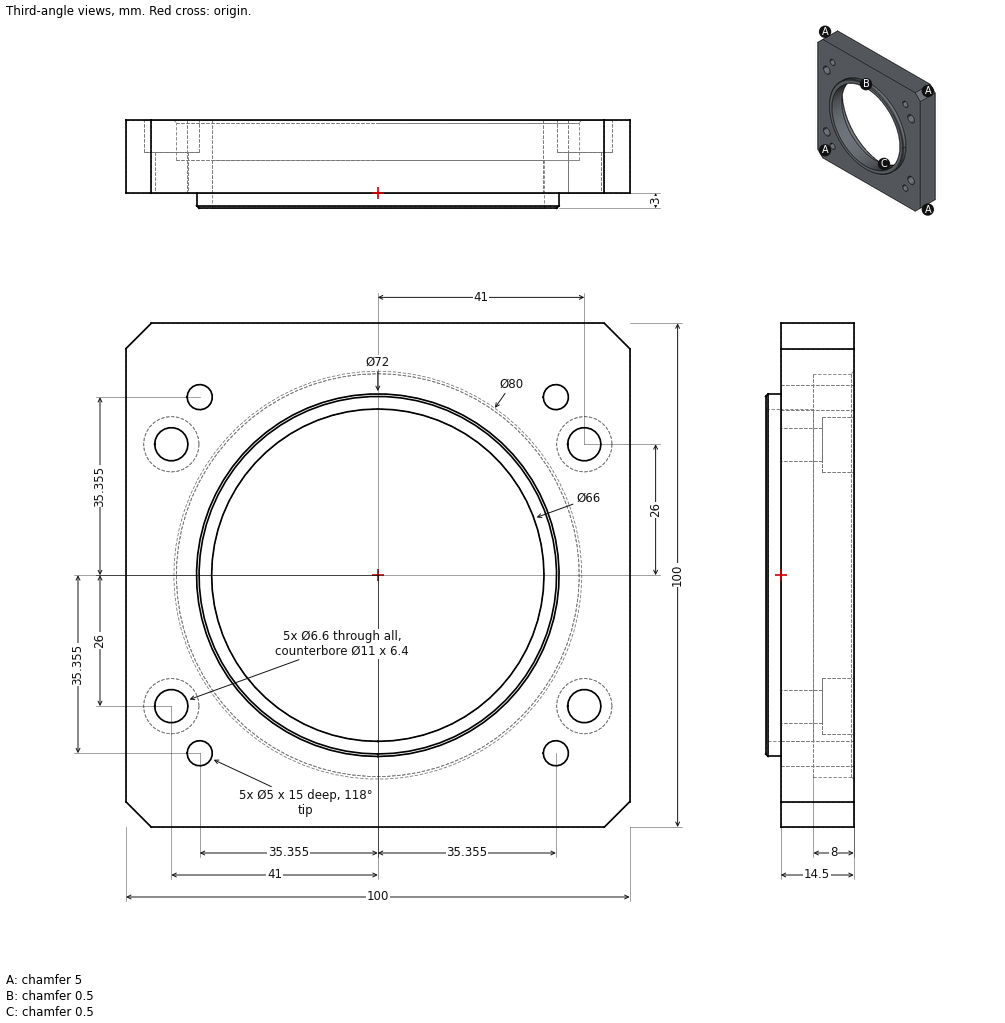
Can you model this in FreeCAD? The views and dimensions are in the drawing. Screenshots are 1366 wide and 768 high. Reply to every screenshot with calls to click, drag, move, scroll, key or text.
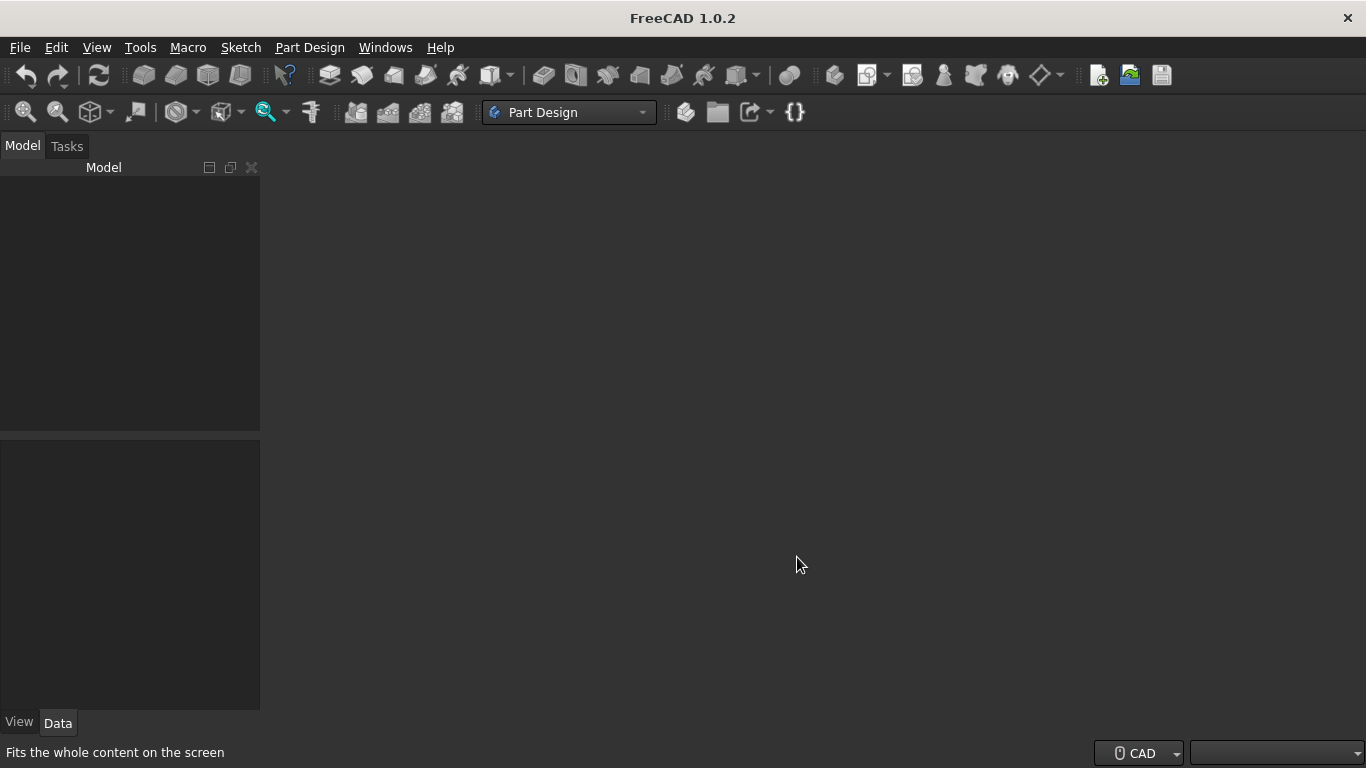
click(1098, 76)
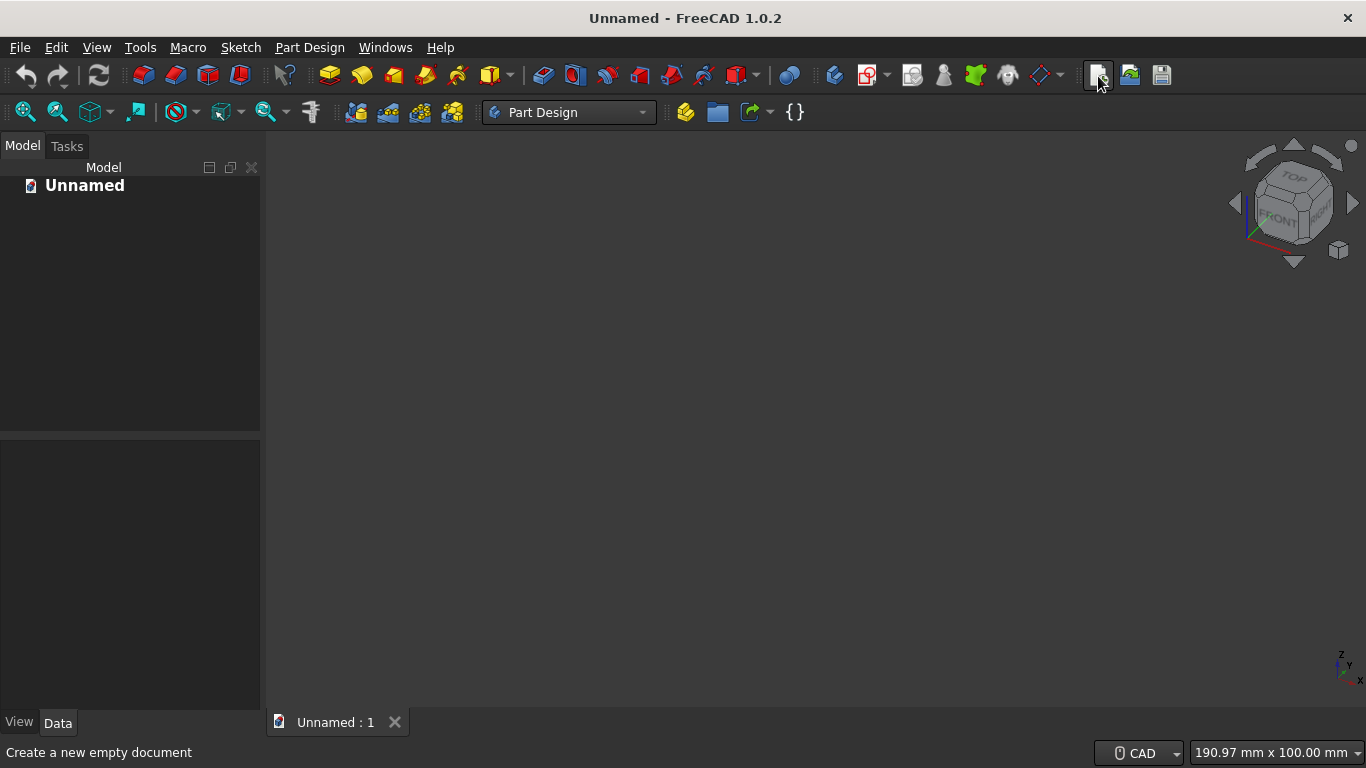
click(868, 76)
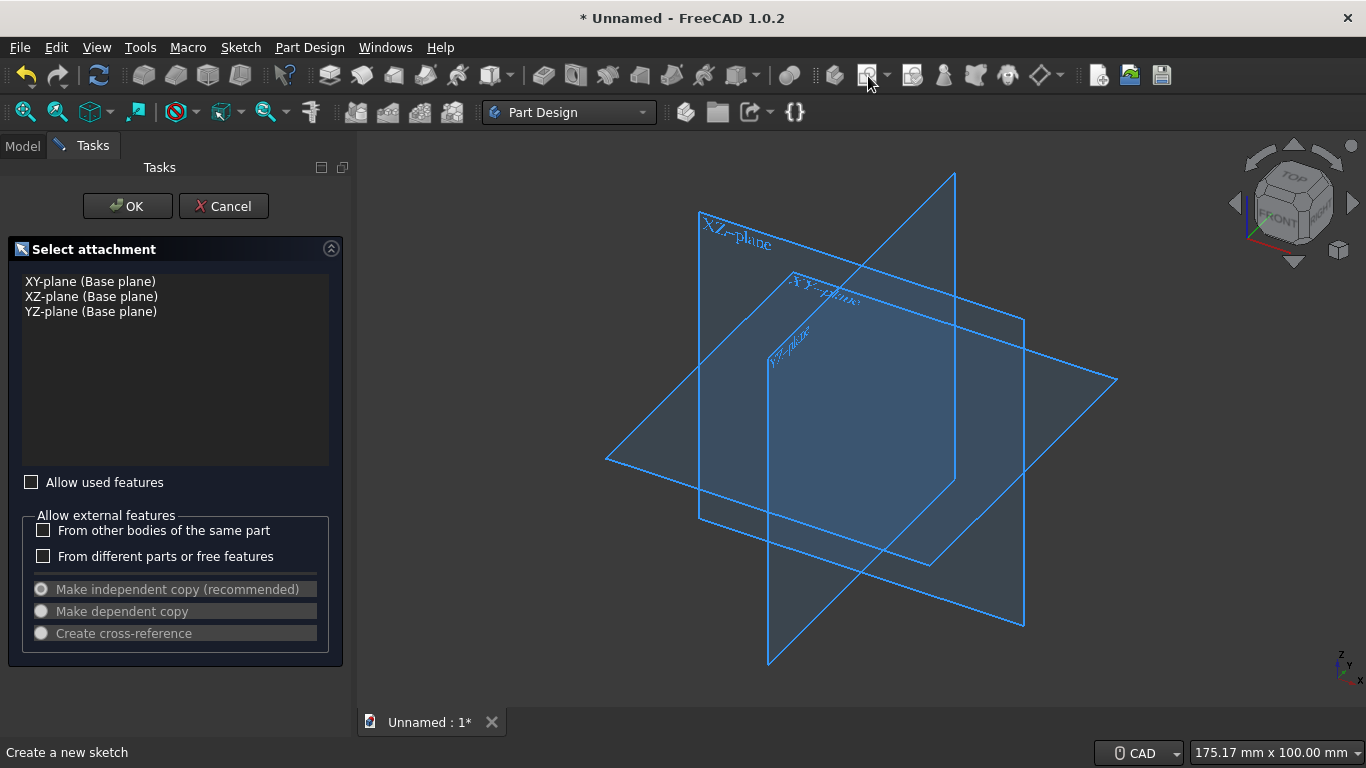
click(82, 296)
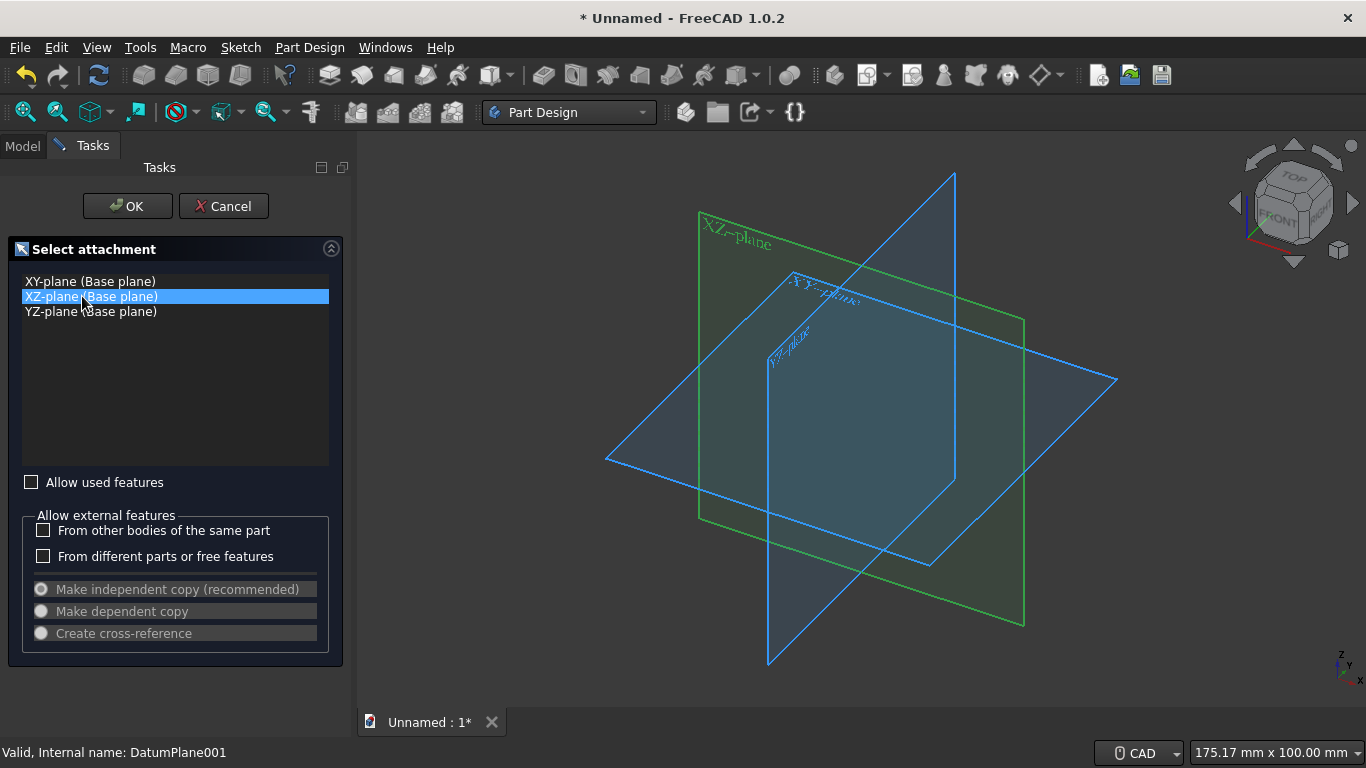
click(128, 206)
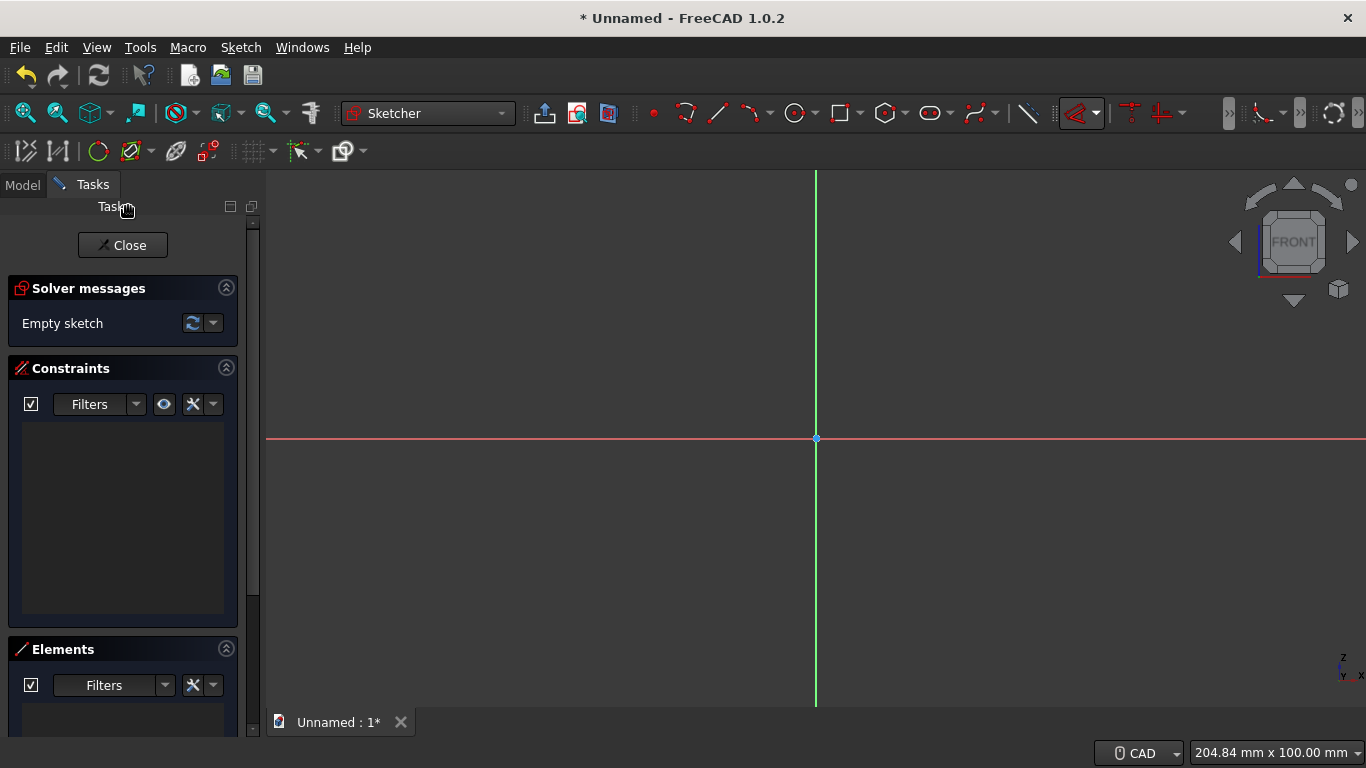
scroll(608, 438, down, 2)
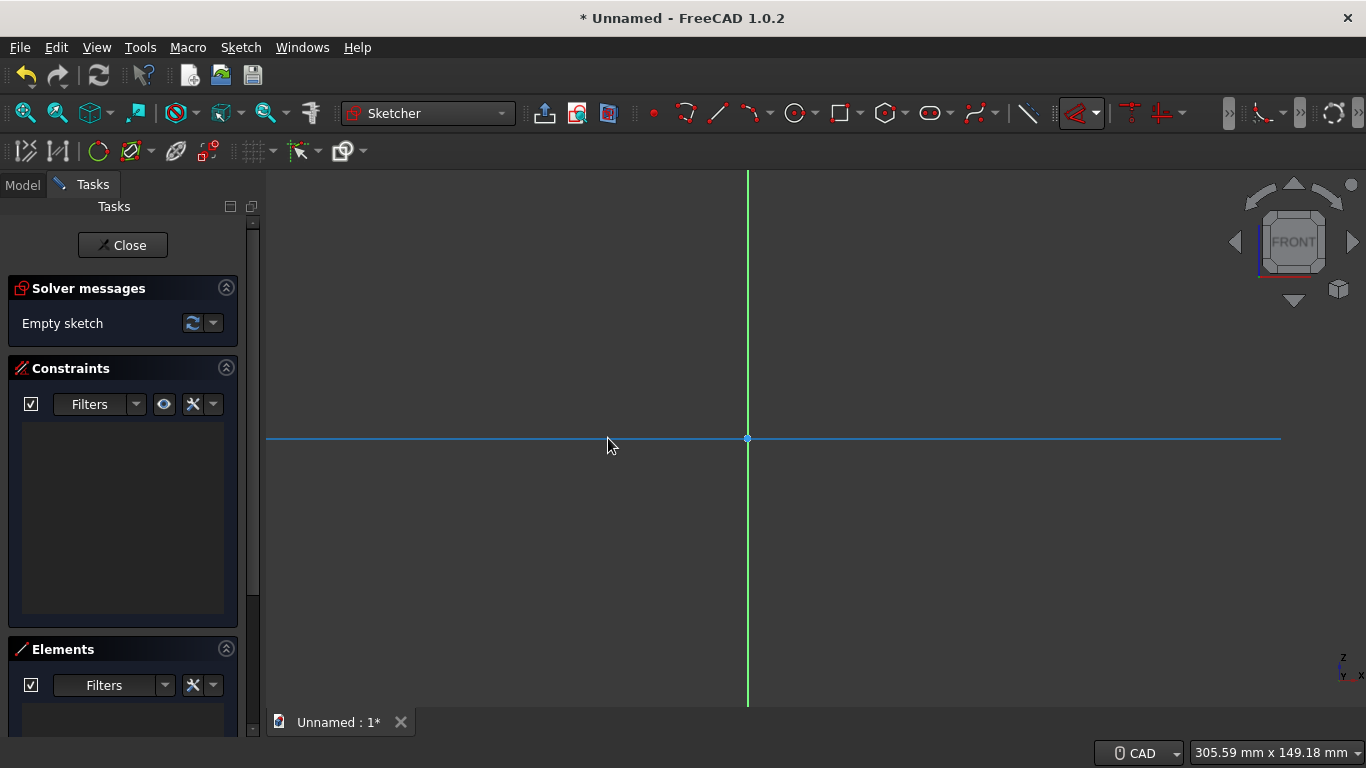
key(g)
key(v)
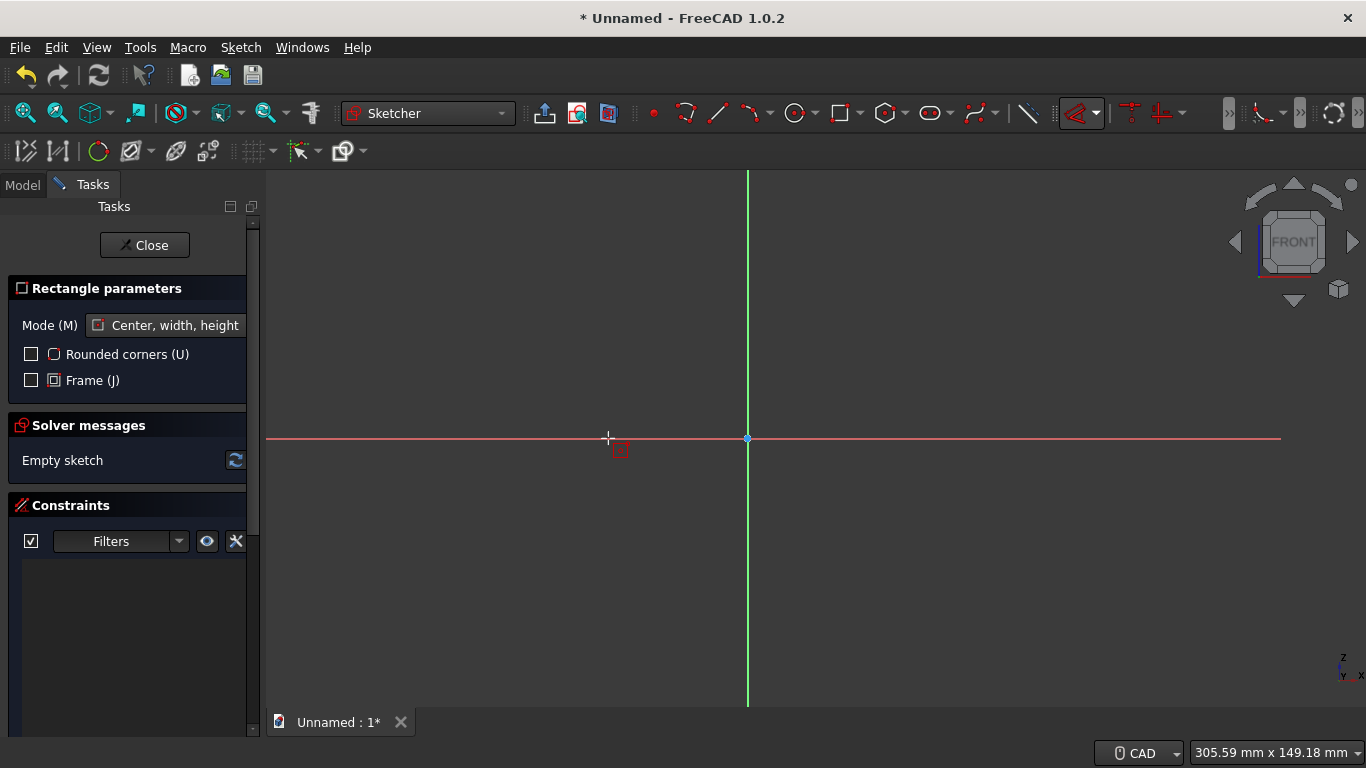
click(748, 438)
click(928, 259)
key(Escape)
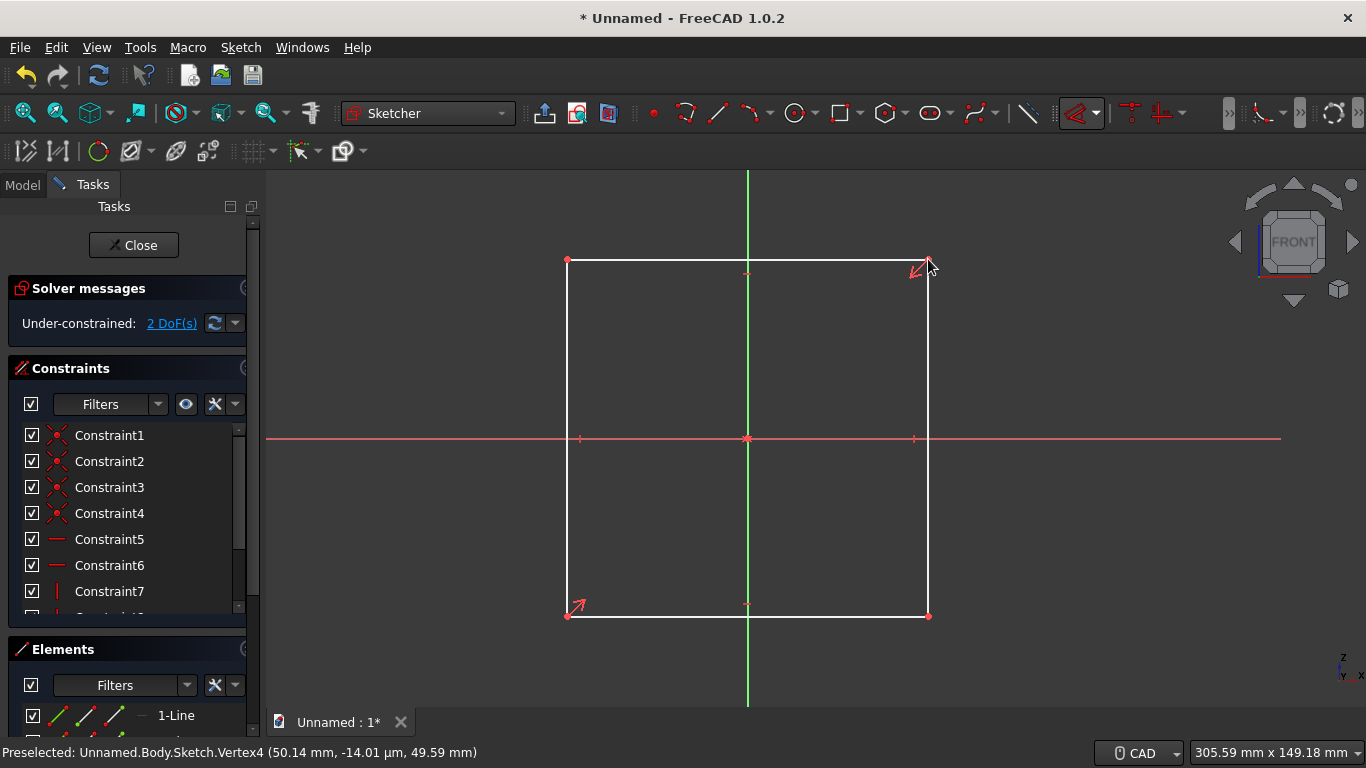
key(d)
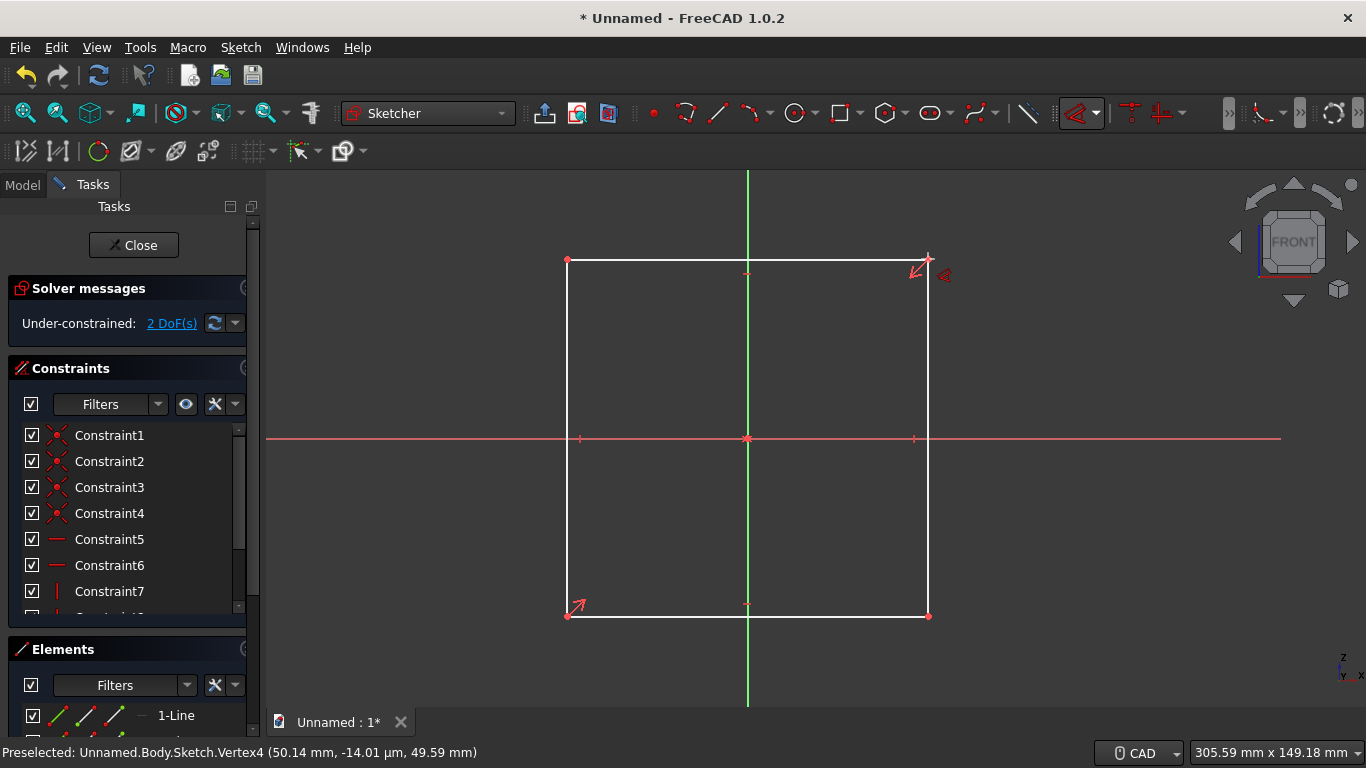
click(675, 617)
click(665, 651)